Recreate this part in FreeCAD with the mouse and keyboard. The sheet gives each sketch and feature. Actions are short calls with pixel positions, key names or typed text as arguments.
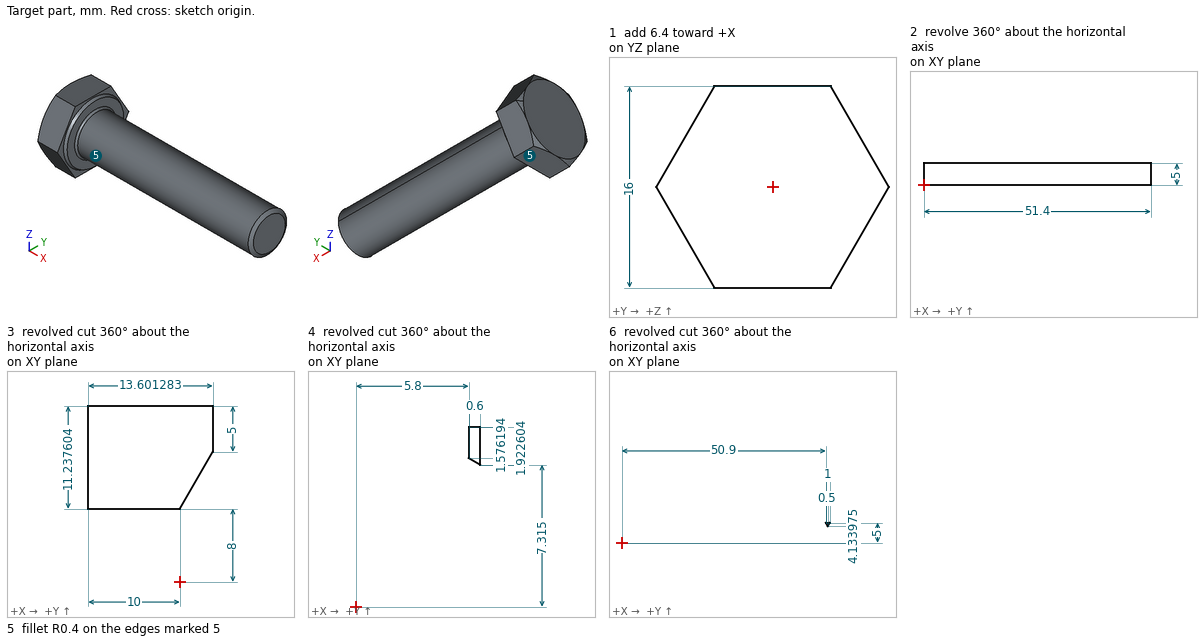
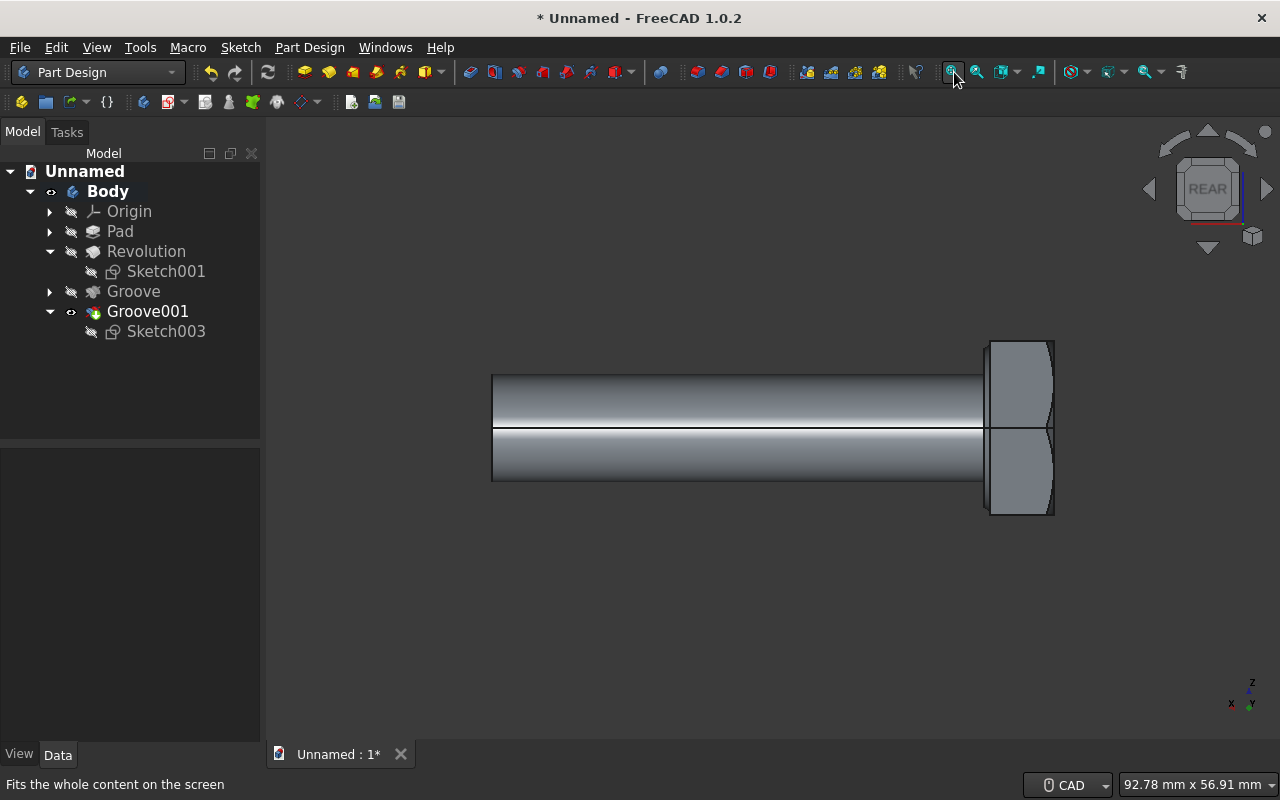
key(6)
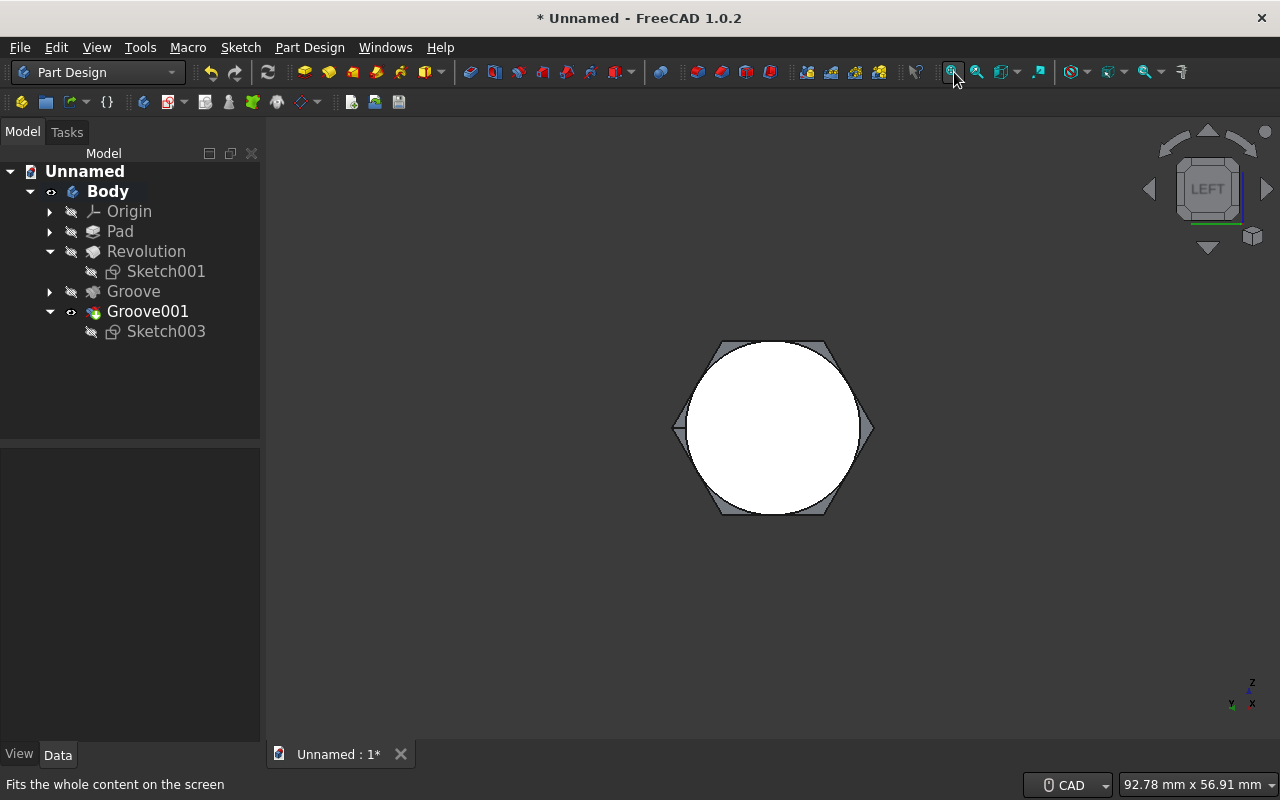
click(954, 72)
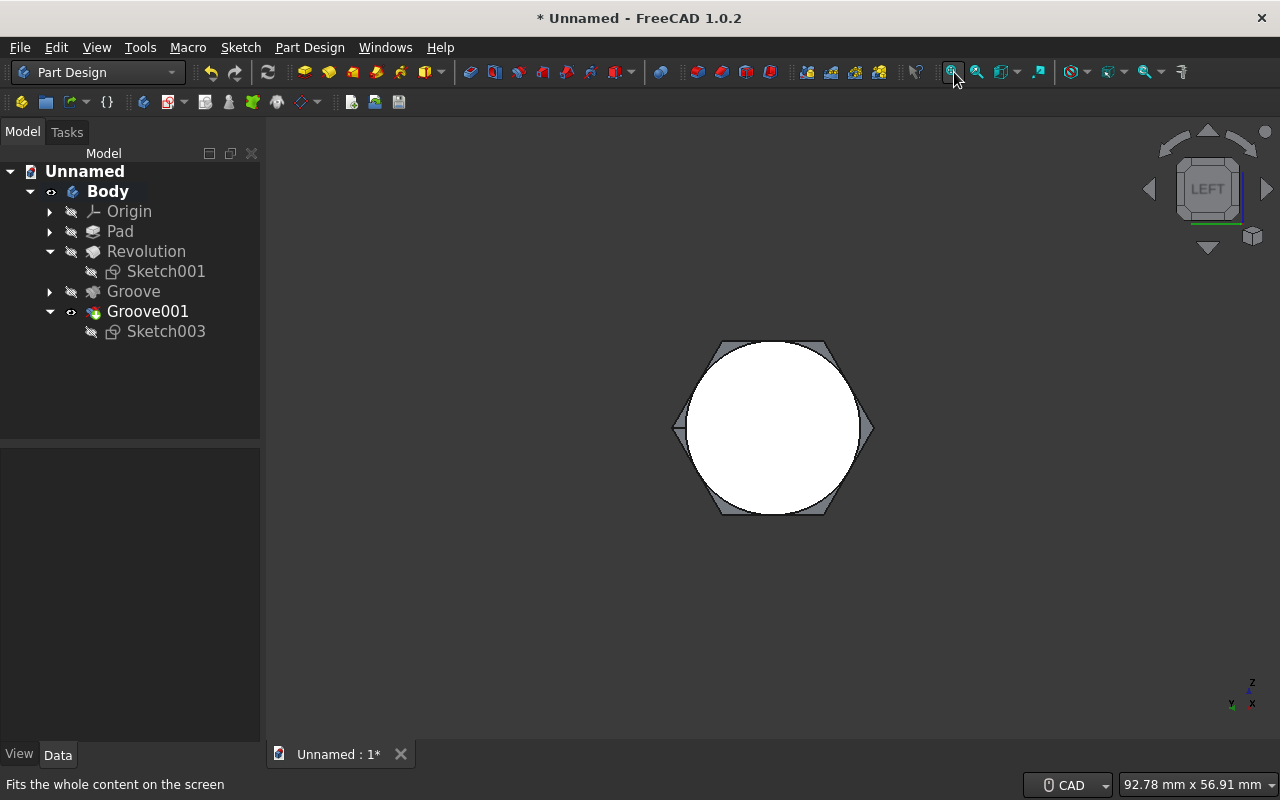
key(v)
key(3)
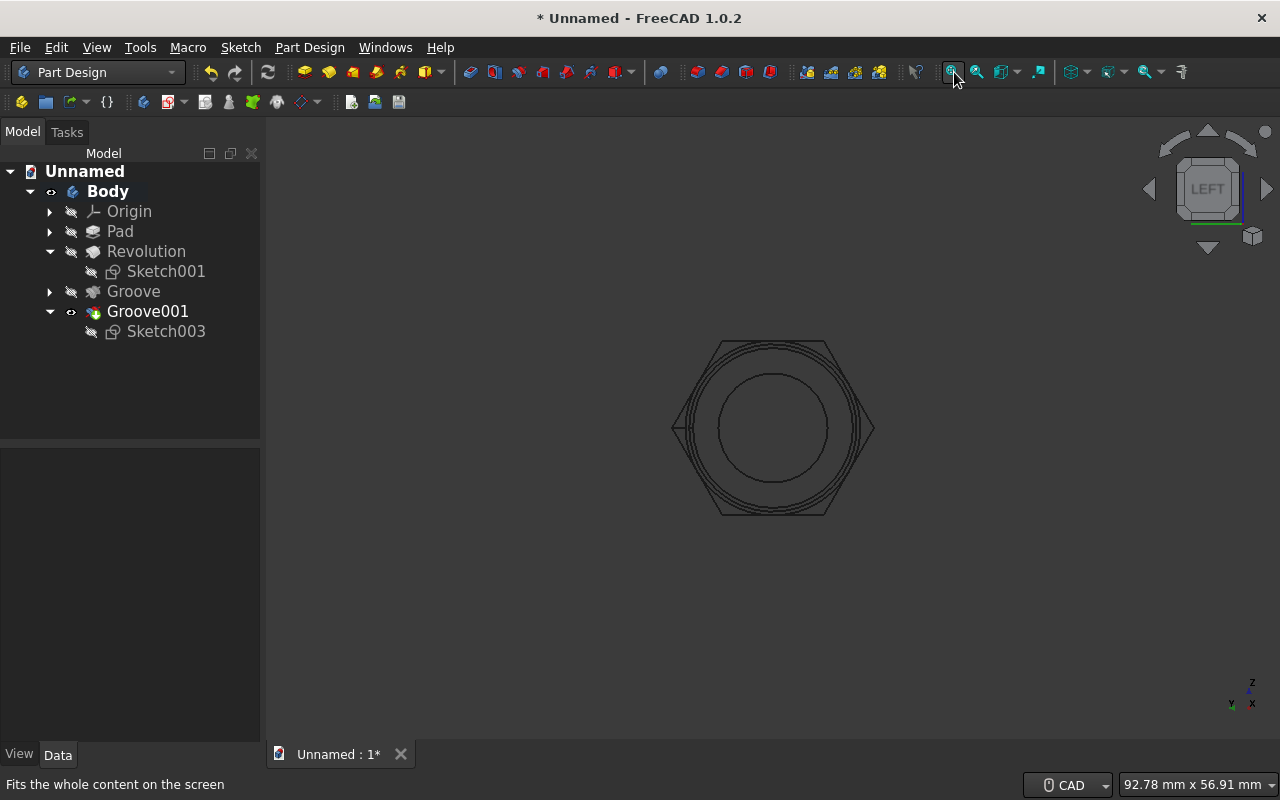
key(0)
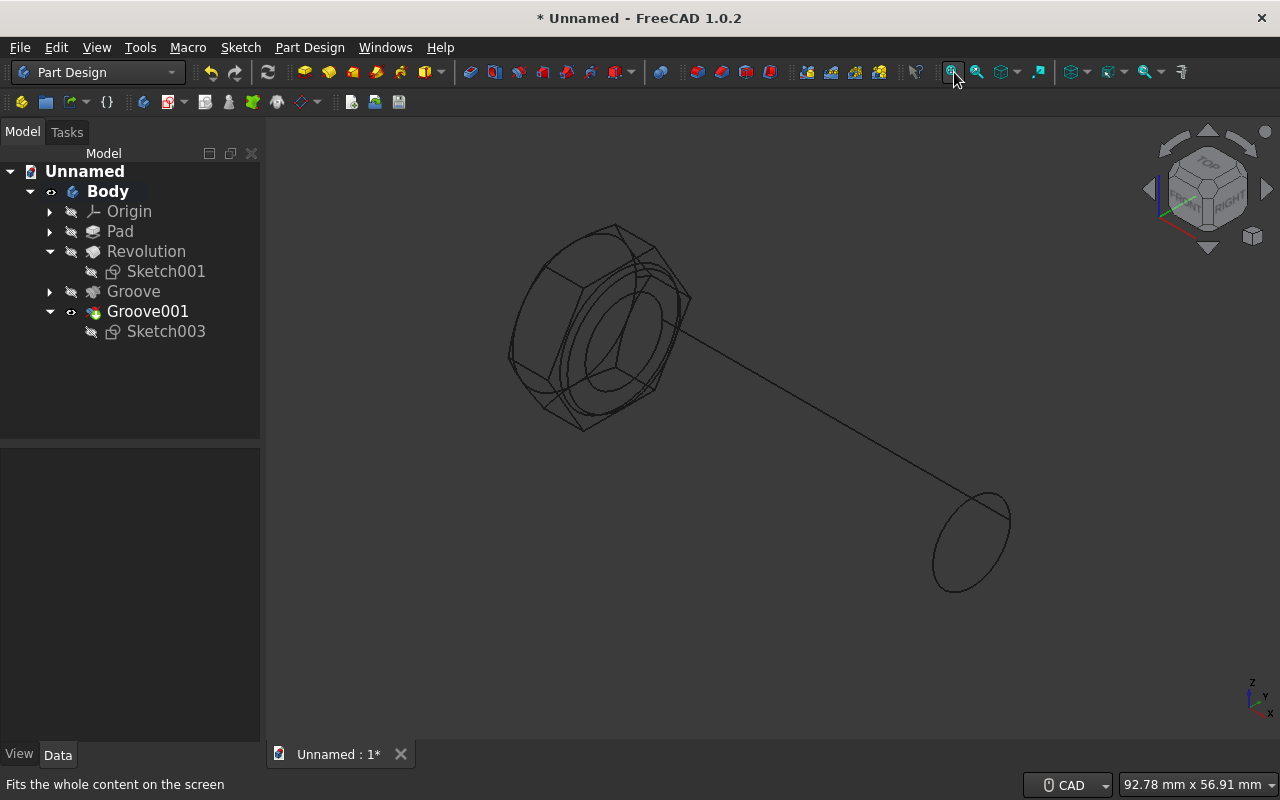
click(585, 363)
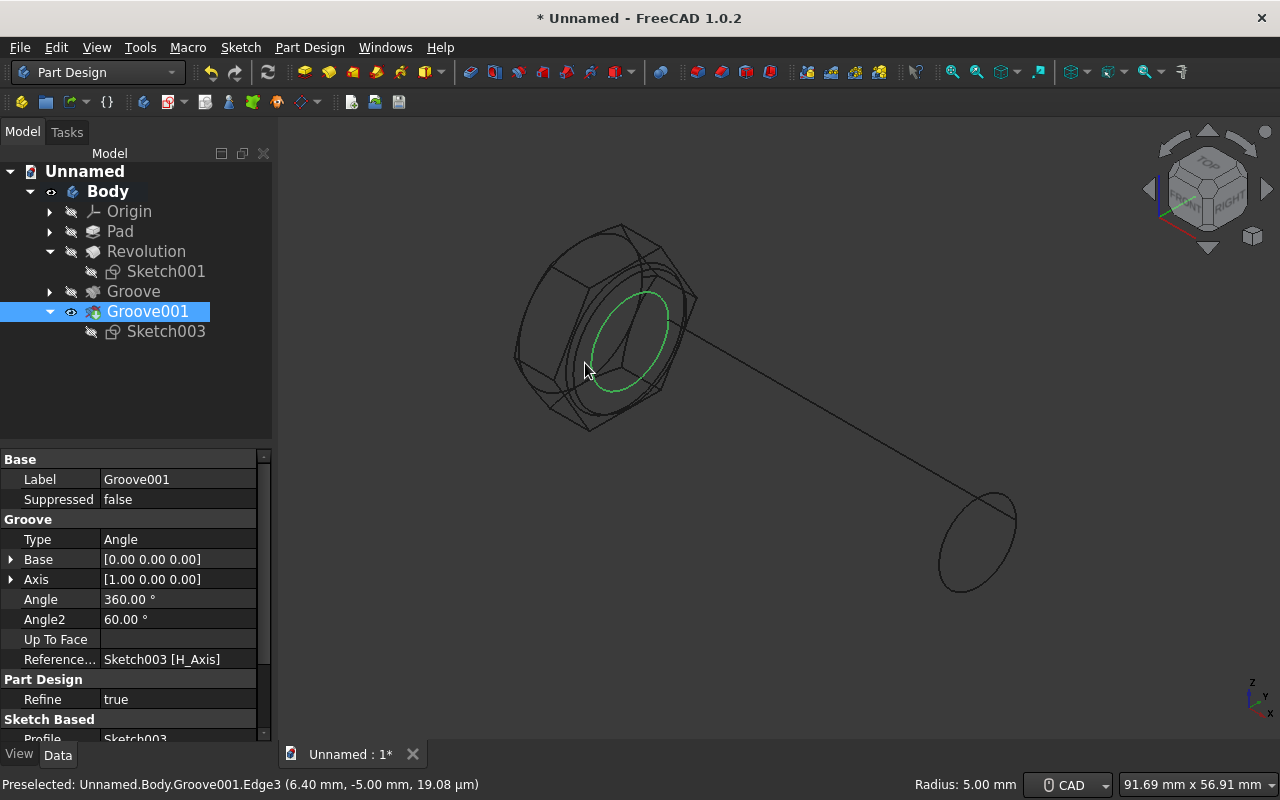
key(v)
key(1)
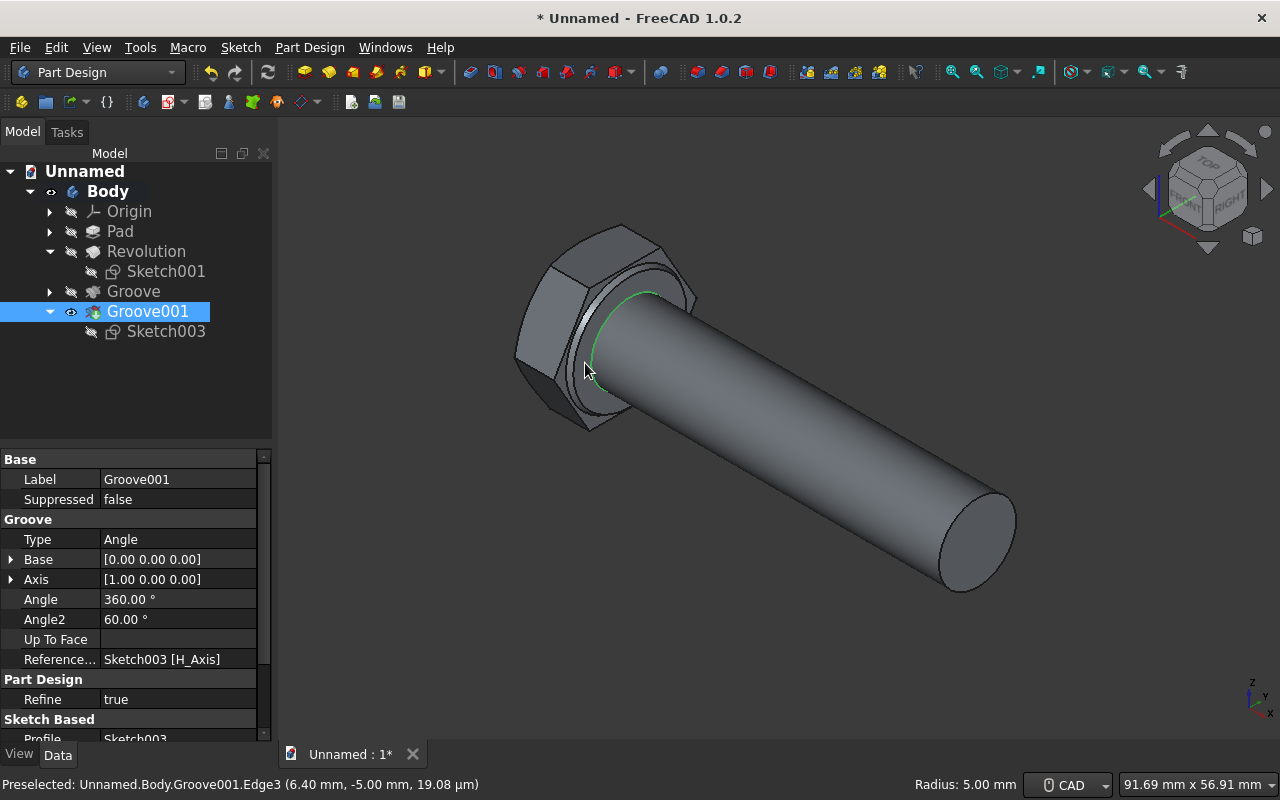
click(698, 72)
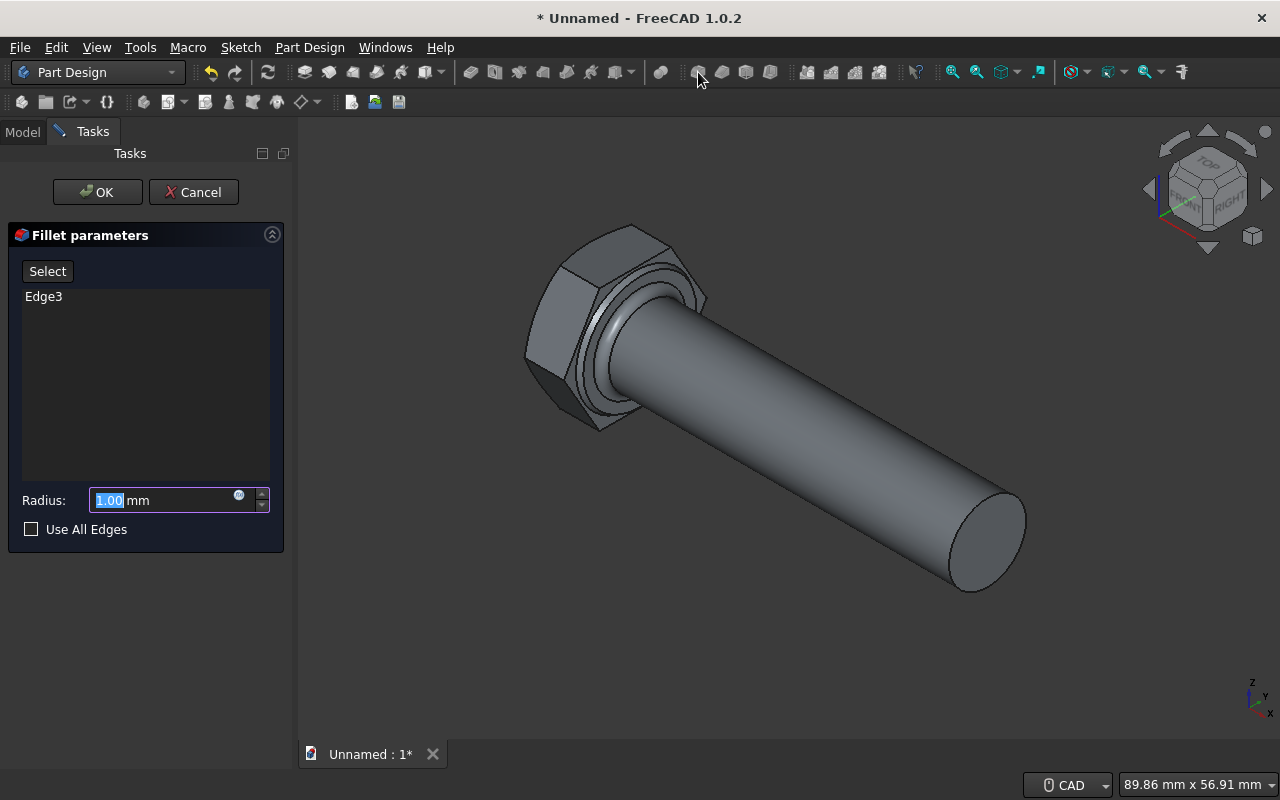
text(0.4)
key(Tab)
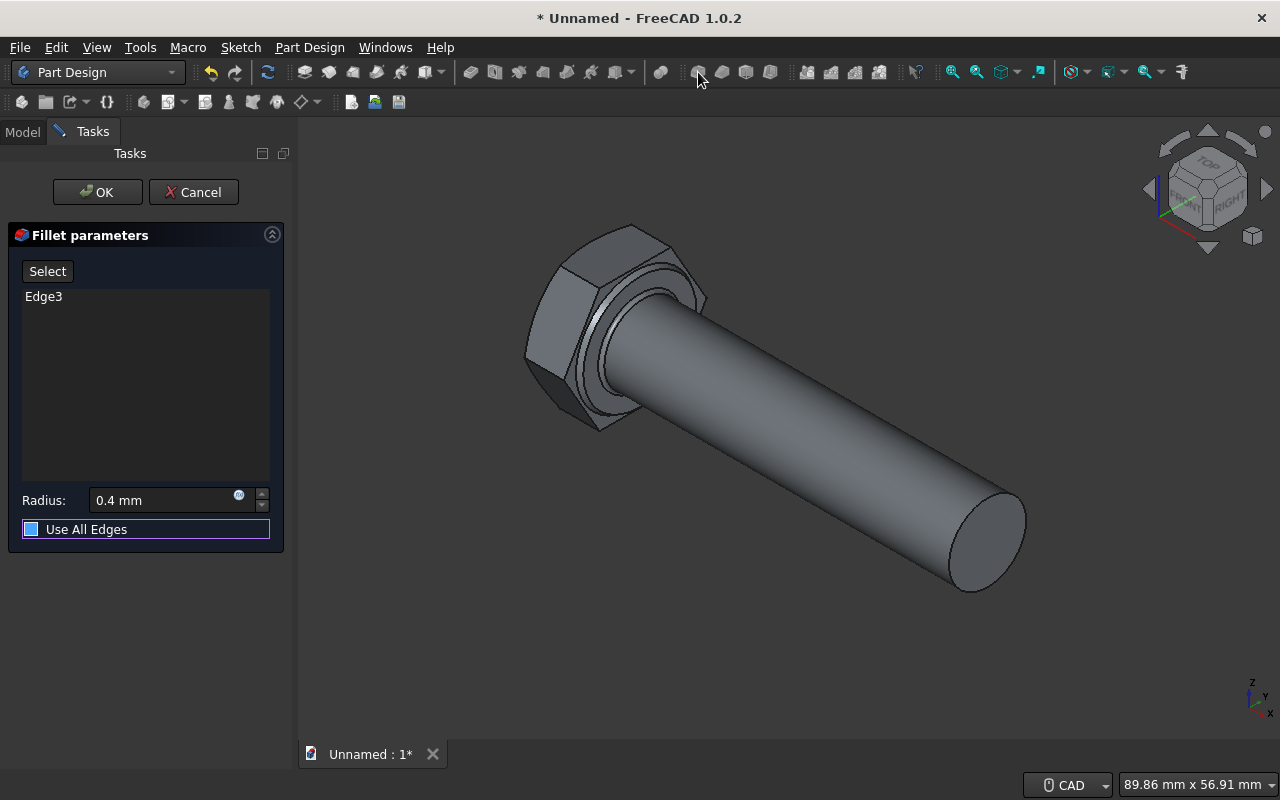
click(98, 192)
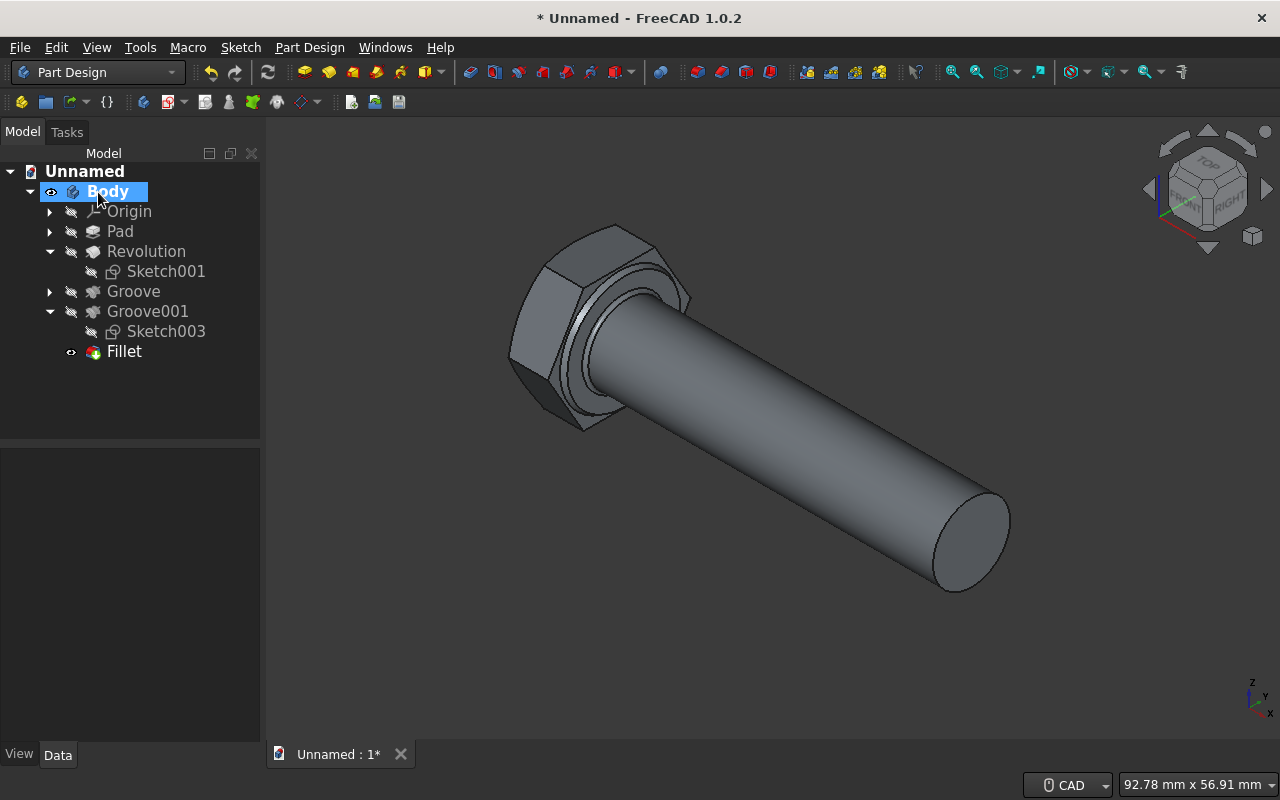
click(168, 102)